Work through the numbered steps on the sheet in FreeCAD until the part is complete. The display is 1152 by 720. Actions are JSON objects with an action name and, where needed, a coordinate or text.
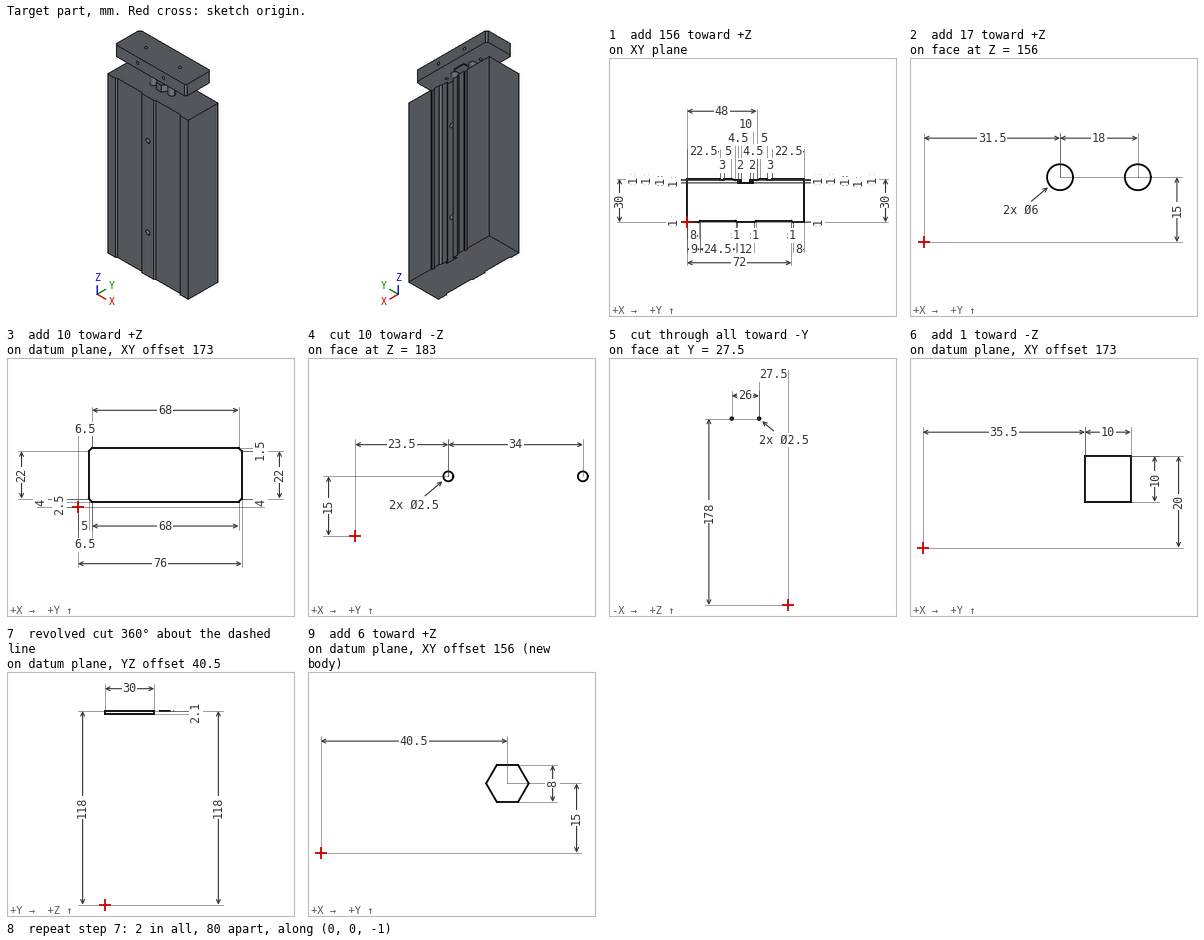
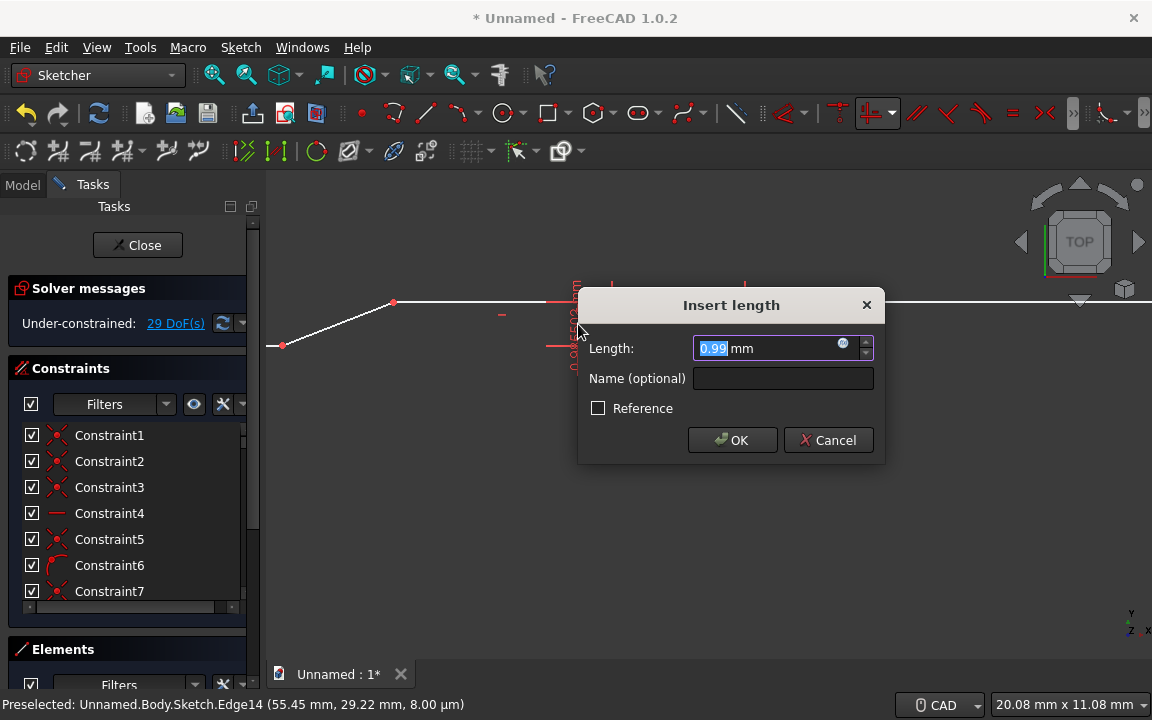
{"action": "type", "text": "1"}
{"action": "key", "text": "Return"}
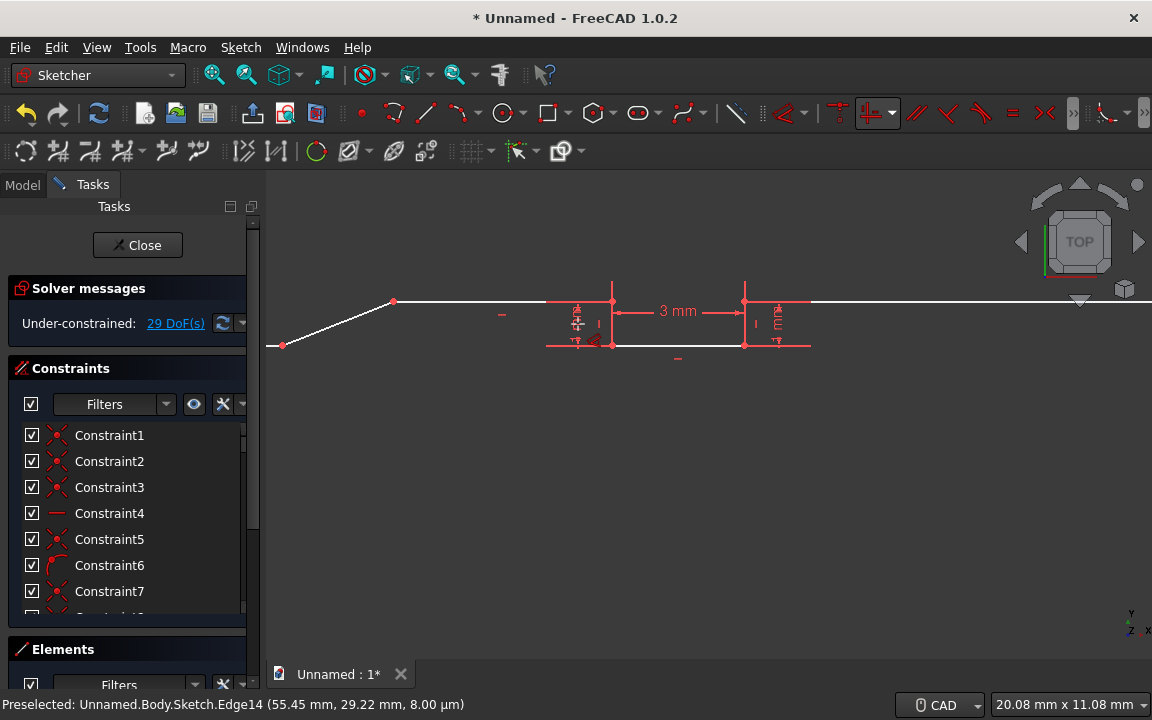
{"action": "scroll", "coordinate": [748, 329], "scroll_direction": "down", "scroll_amount": 10}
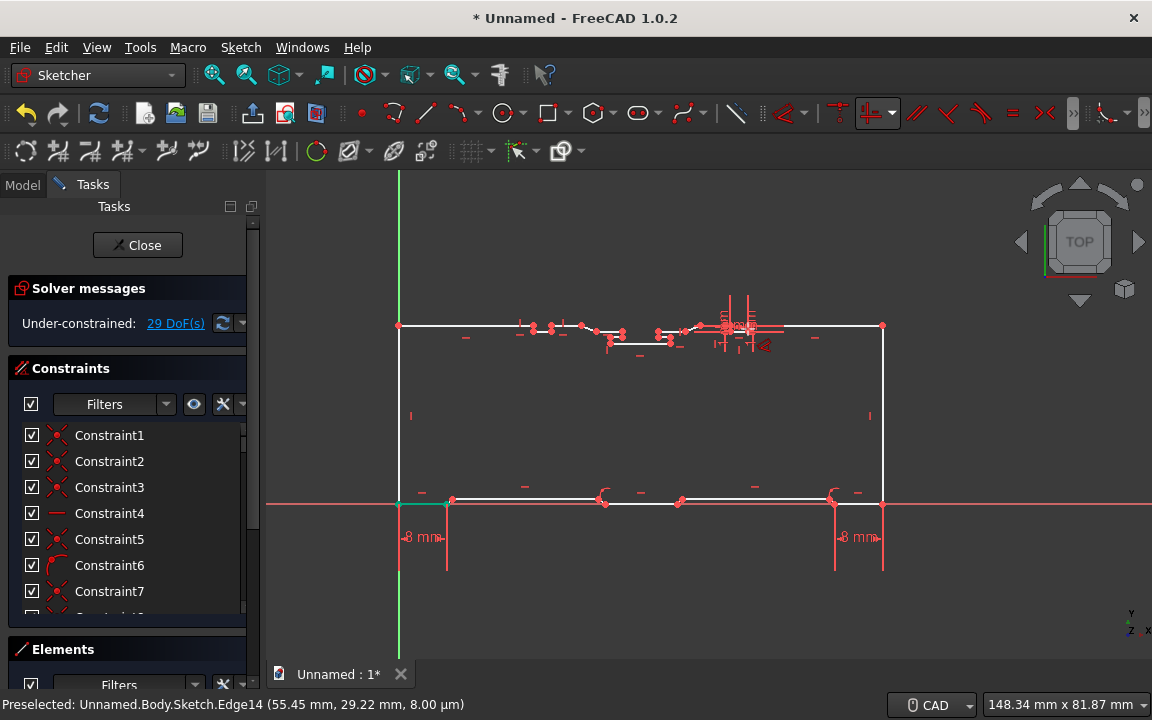
{"action": "scroll", "coordinate": [721, 326], "scroll_direction": "up", "scroll_amount": 3}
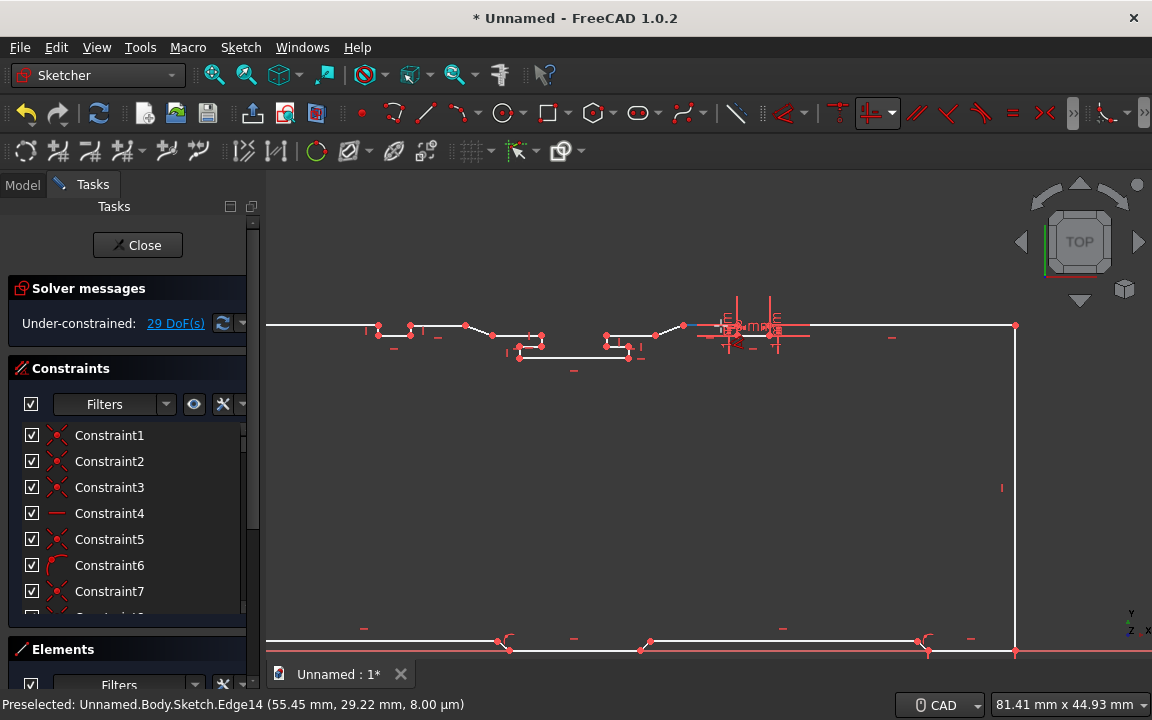
{"action": "left_click", "coordinate": [721, 325]}
{"action": "left_click", "coordinate": [710, 291]}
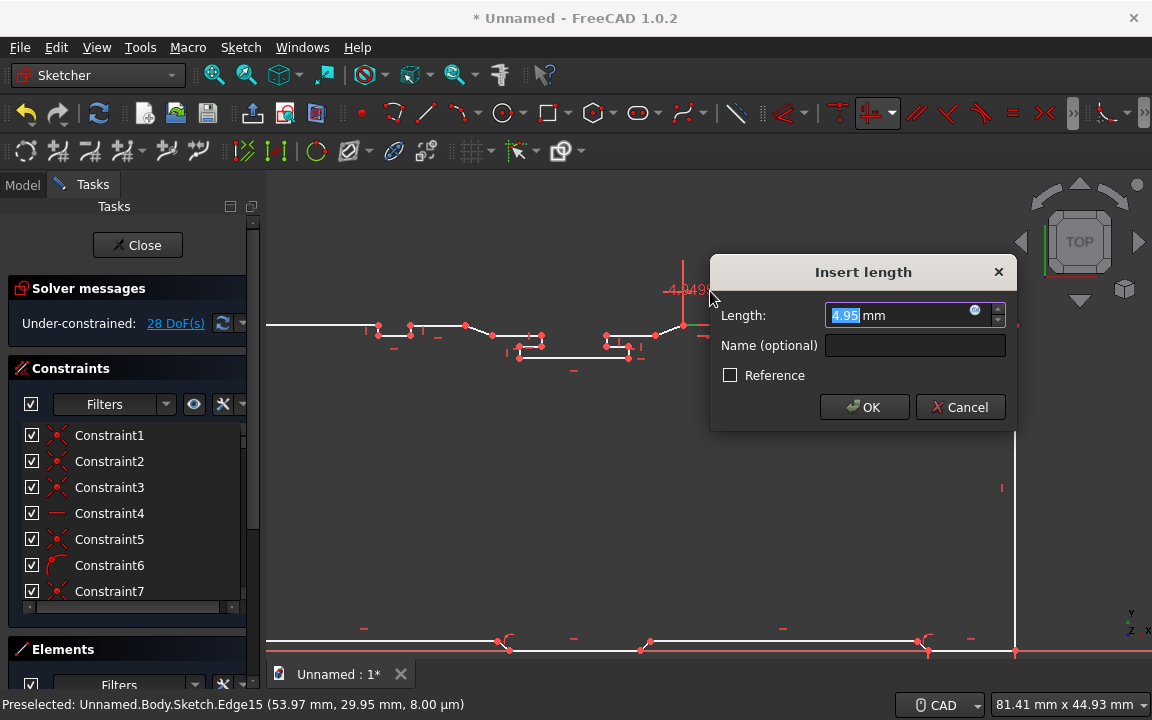
{"action": "type", "text": "5"}
{"action": "key", "text": "Return"}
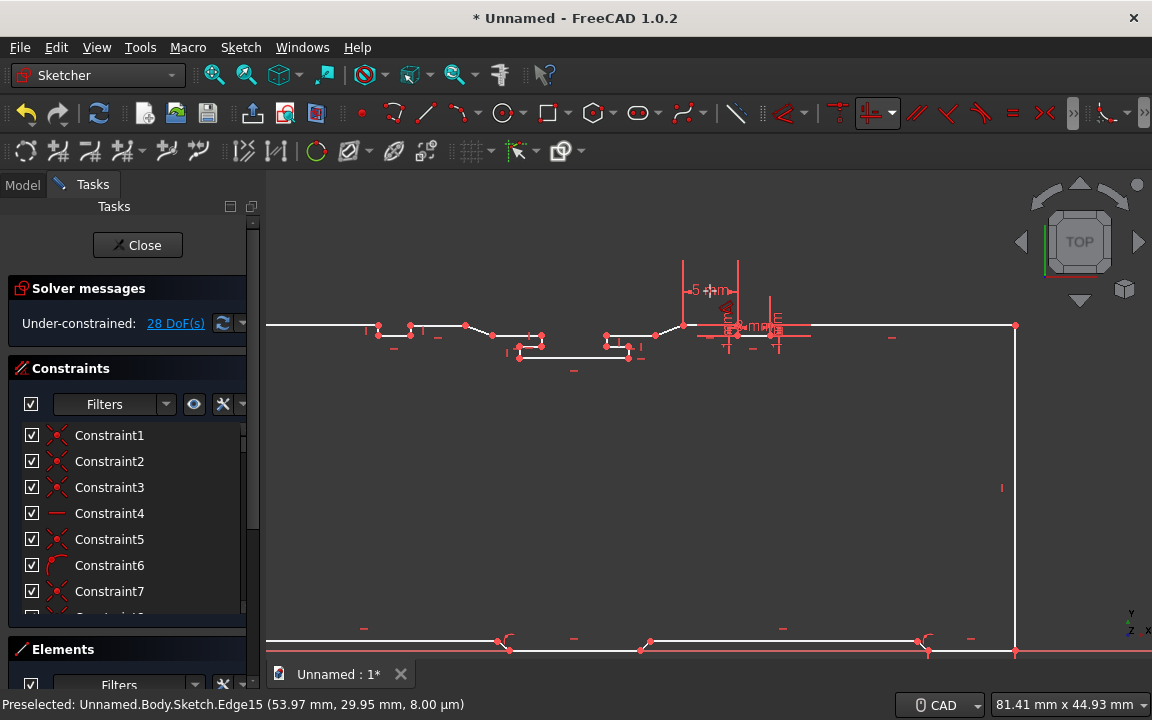
{"action": "scroll", "coordinate": [607, 341], "scroll_direction": "up", "scroll_amount": 7}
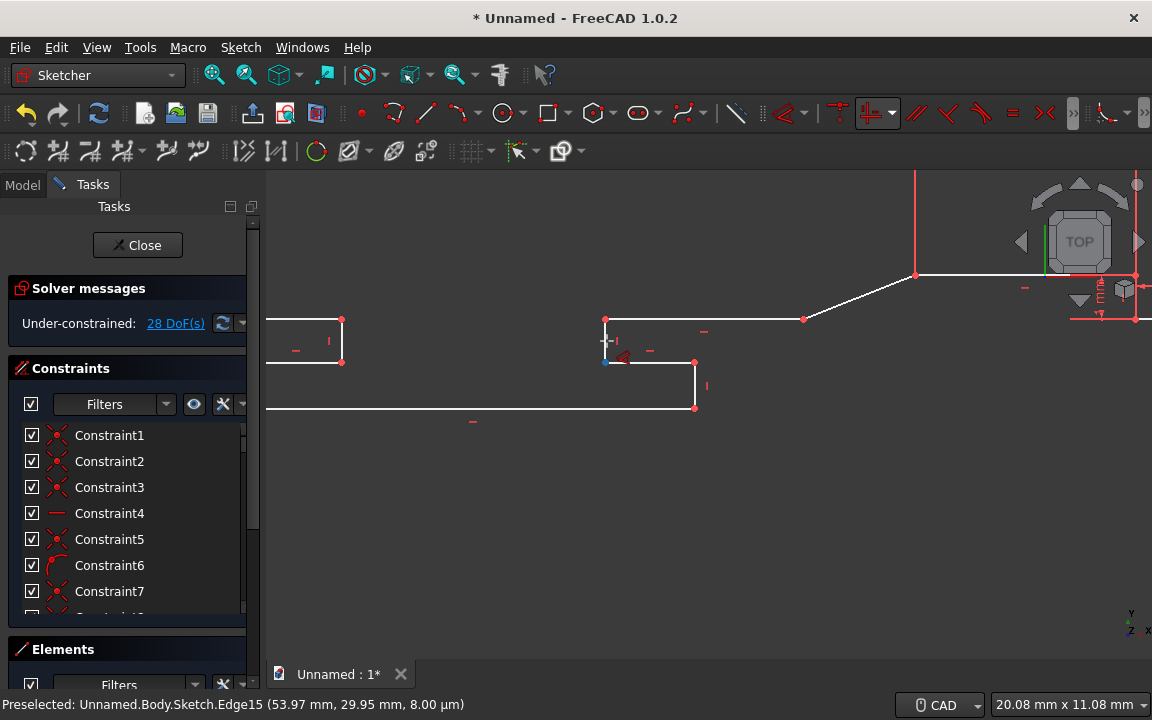
{"action": "left_click", "coordinate": [605, 341]}
{"action": "left_click", "coordinate": [639, 341]}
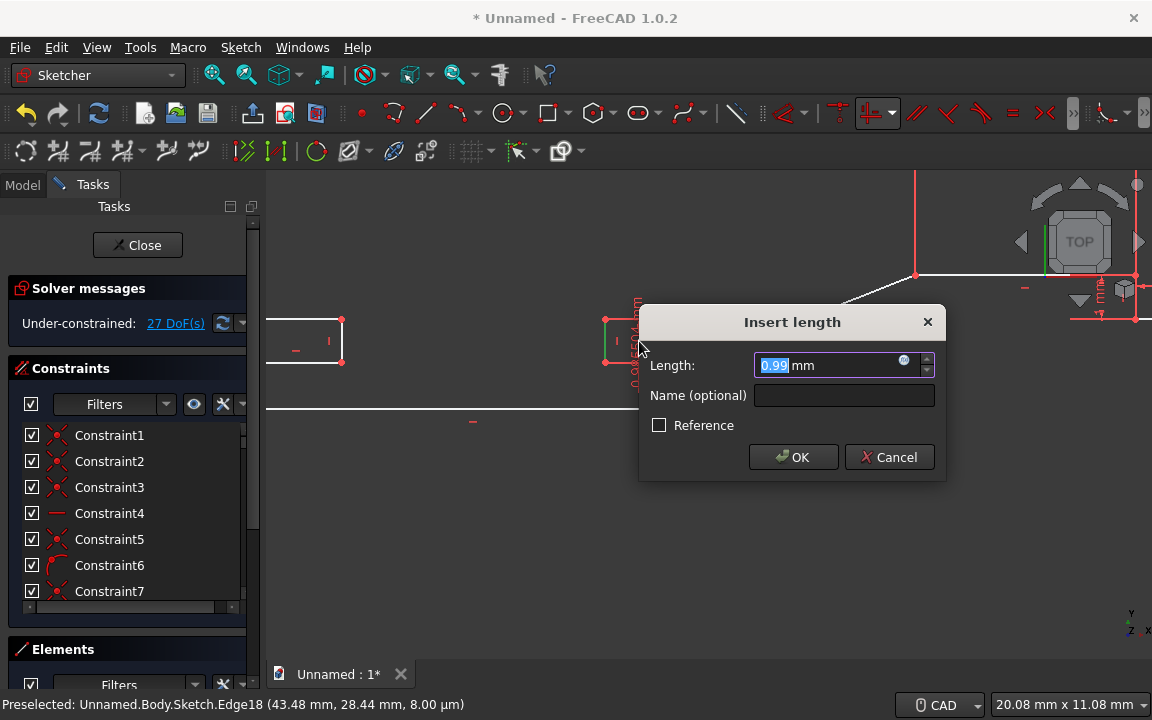
{"action": "type", "text": "1"}
{"action": "key", "text": "Return"}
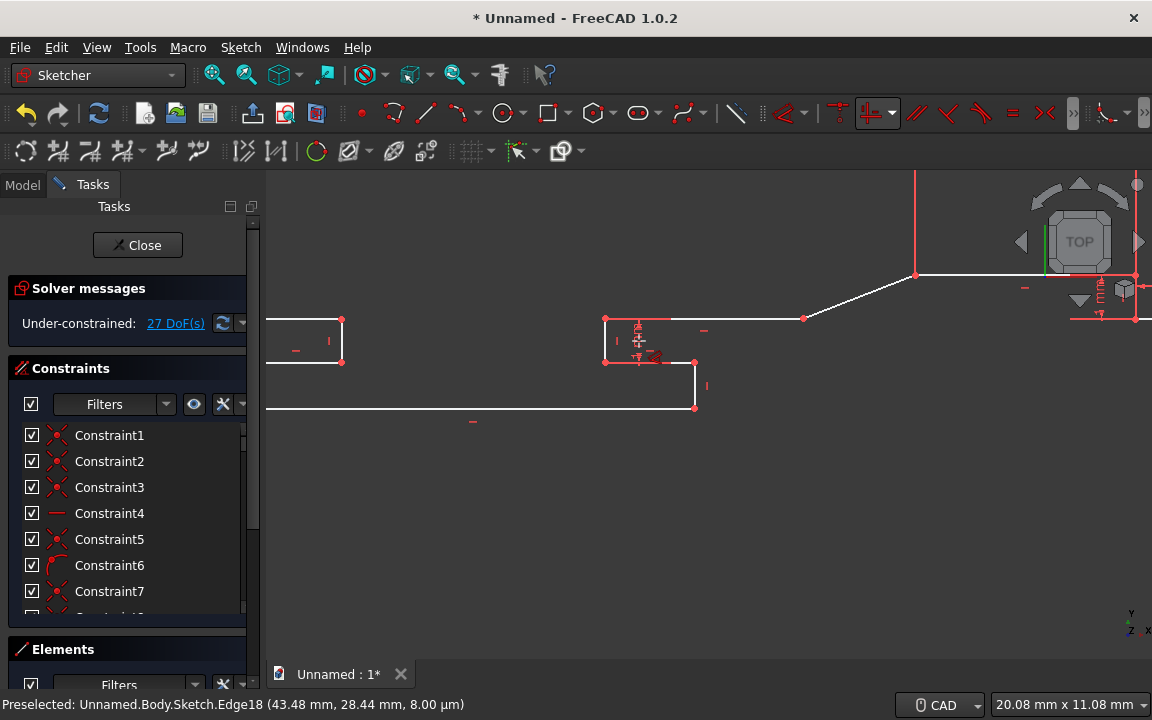
{"action": "left_click", "coordinate": [632, 363]}
{"action": "left_click", "coordinate": [650, 305]}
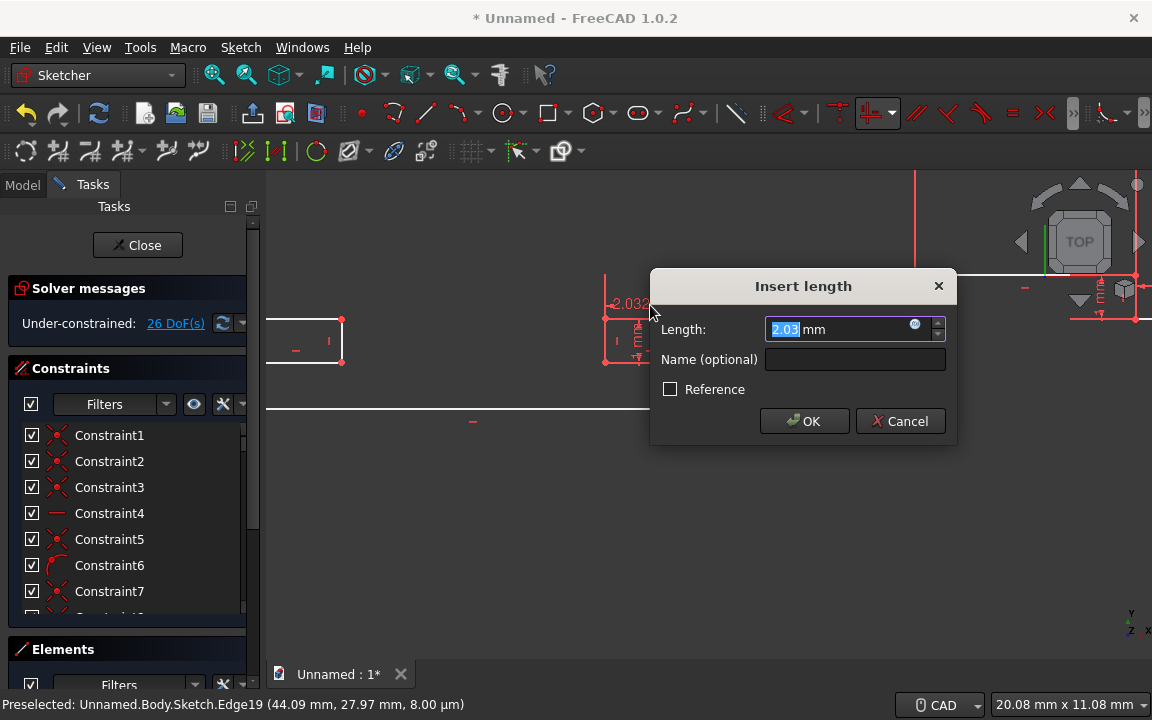
{"action": "type", "text": "2"}
{"action": "key", "text": "Return"}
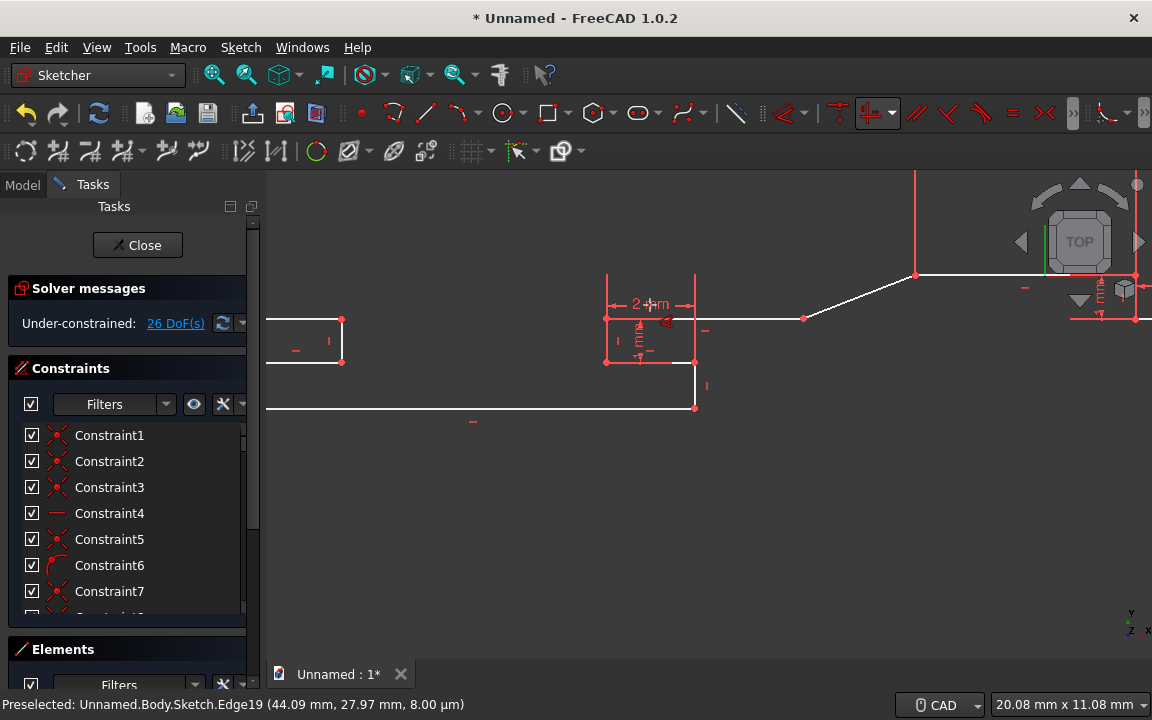
{"action": "left_click", "coordinate": [695, 377]}
{"action": "left_click", "coordinate": [729, 386]}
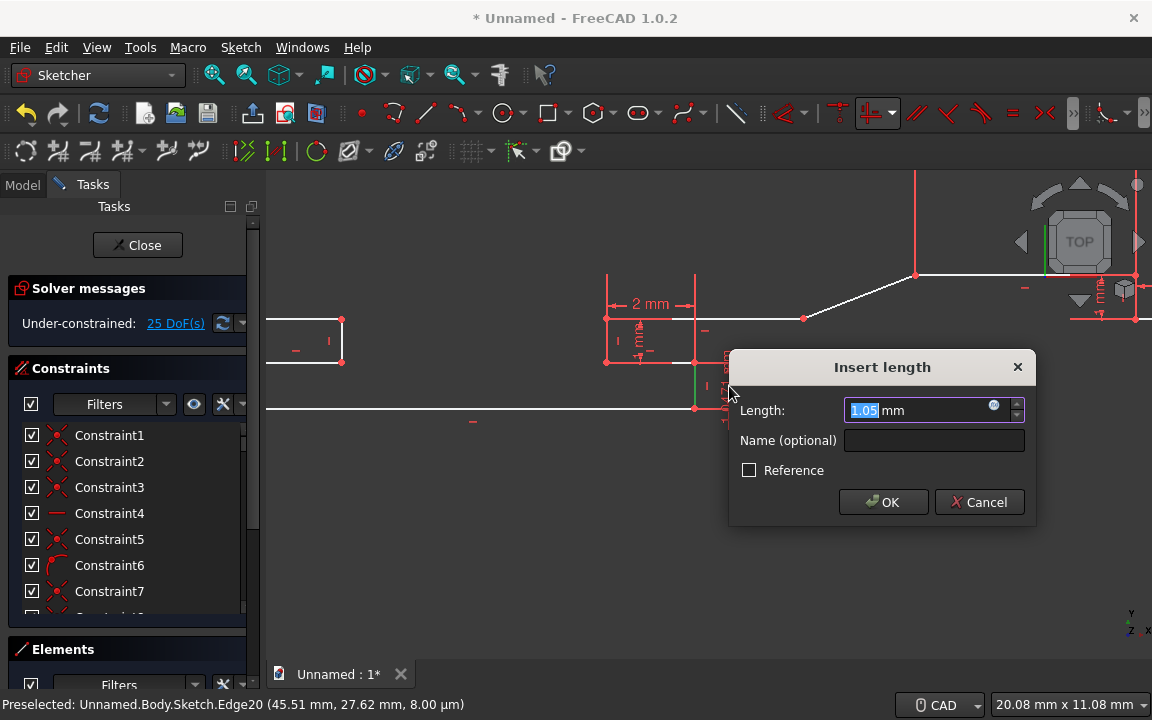
{"action": "type", "text": "1"}
{"action": "key", "text": "Return"}